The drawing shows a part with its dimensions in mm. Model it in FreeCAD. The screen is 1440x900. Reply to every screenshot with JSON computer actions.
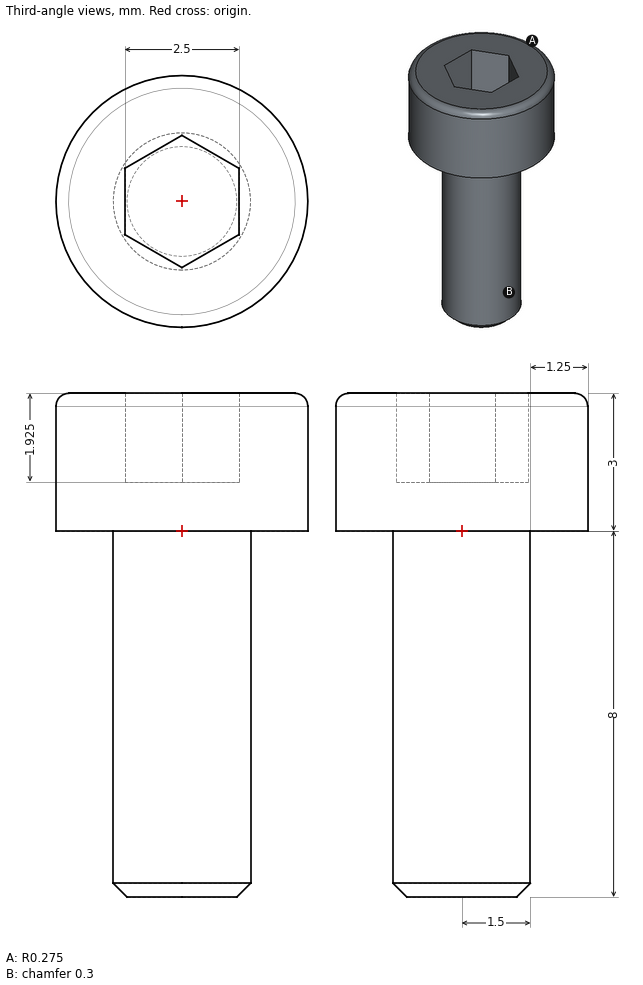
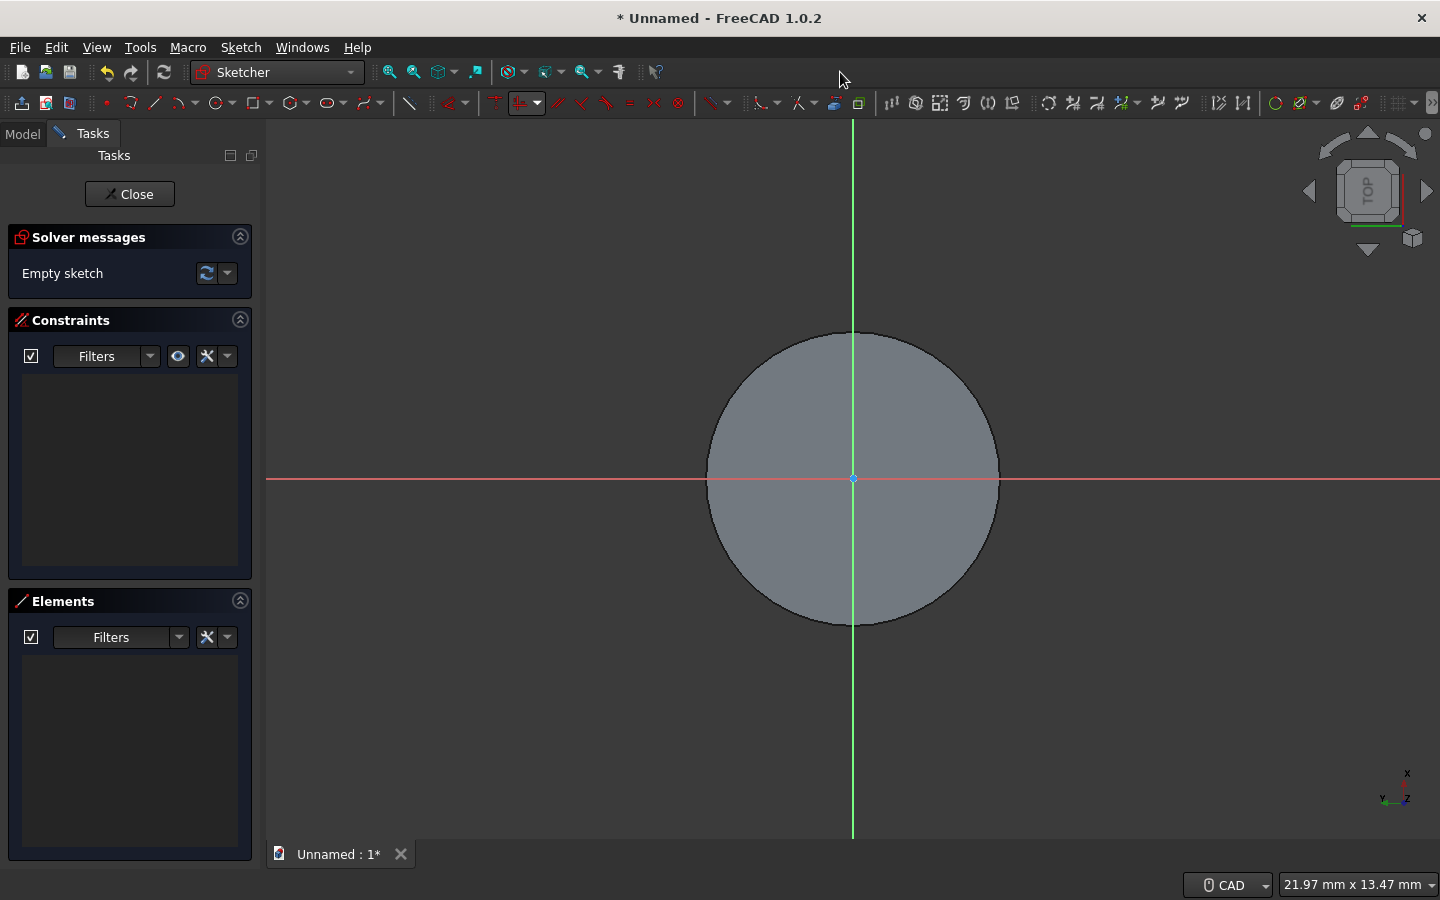
{"action": "scroll", "coordinate": [883, 479], "scroll_direction": "up", "scroll_amount": 6}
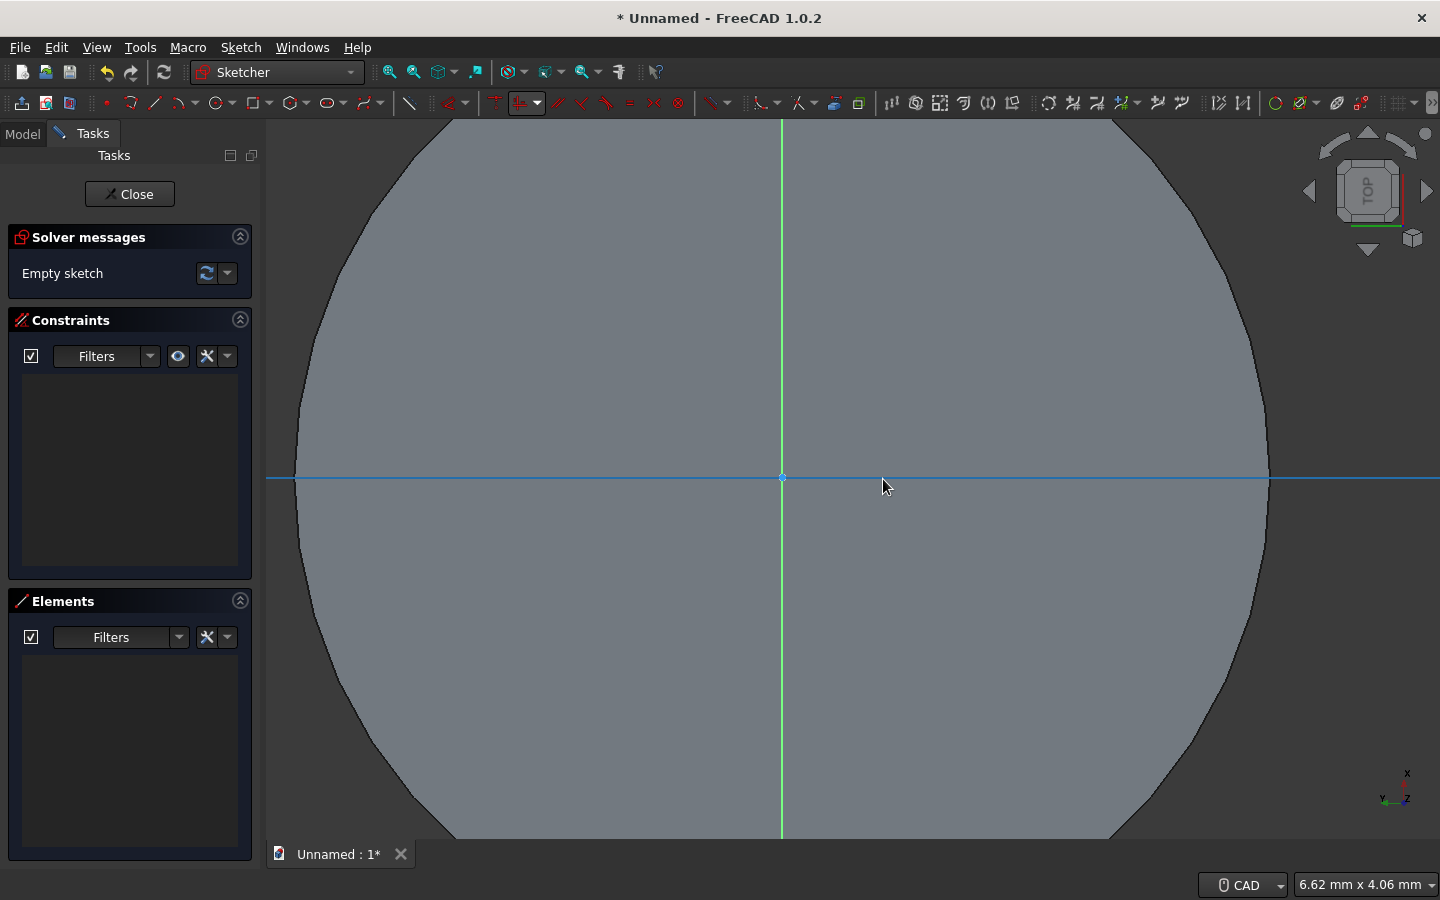
{"action": "left_click", "coordinate": [290, 104]}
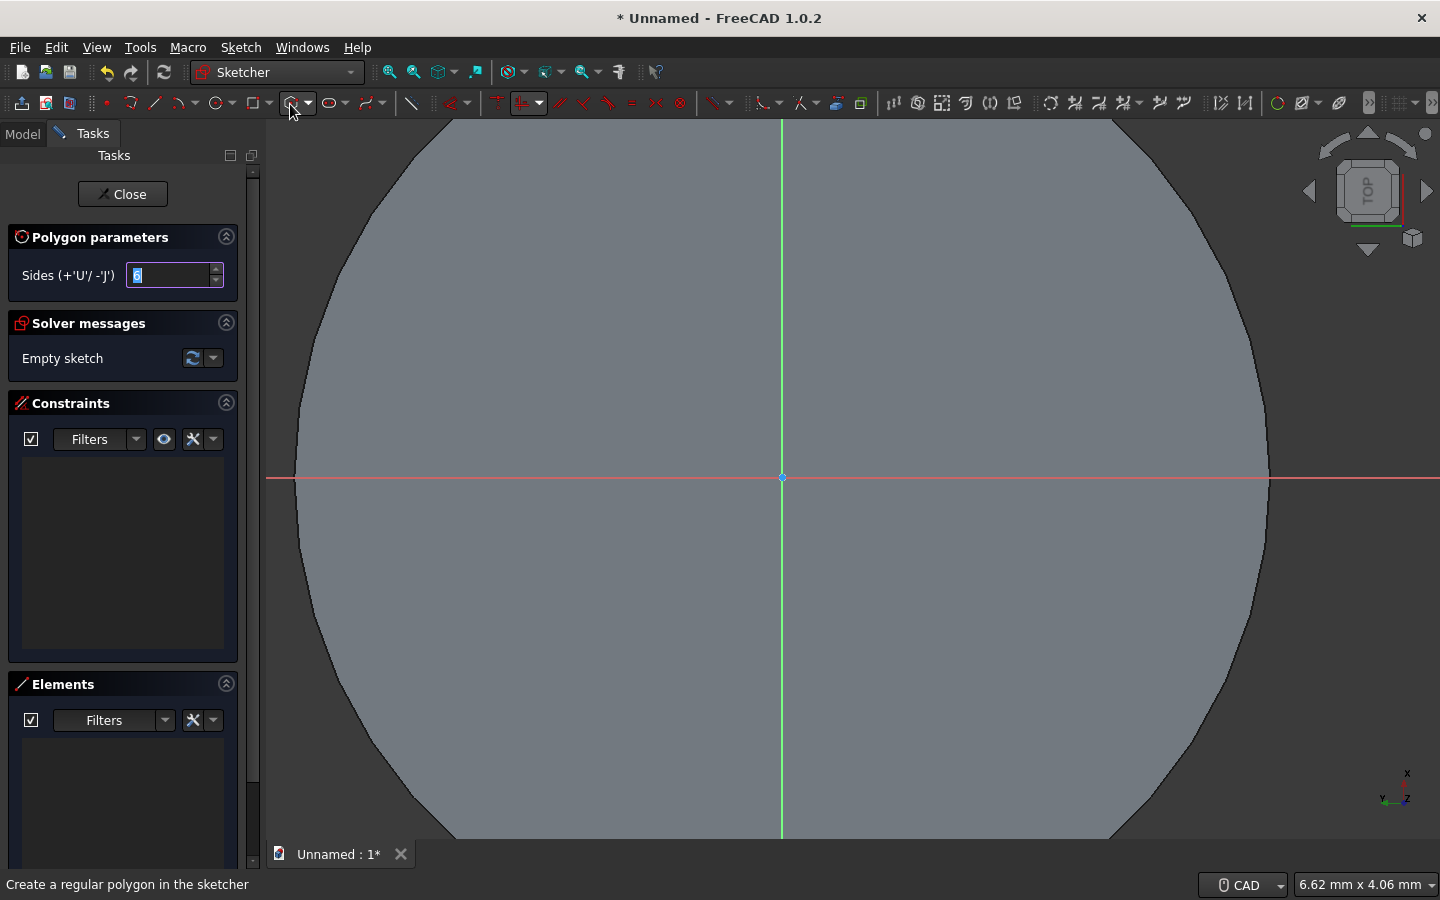
{"action": "left_click", "coordinate": [782, 478]}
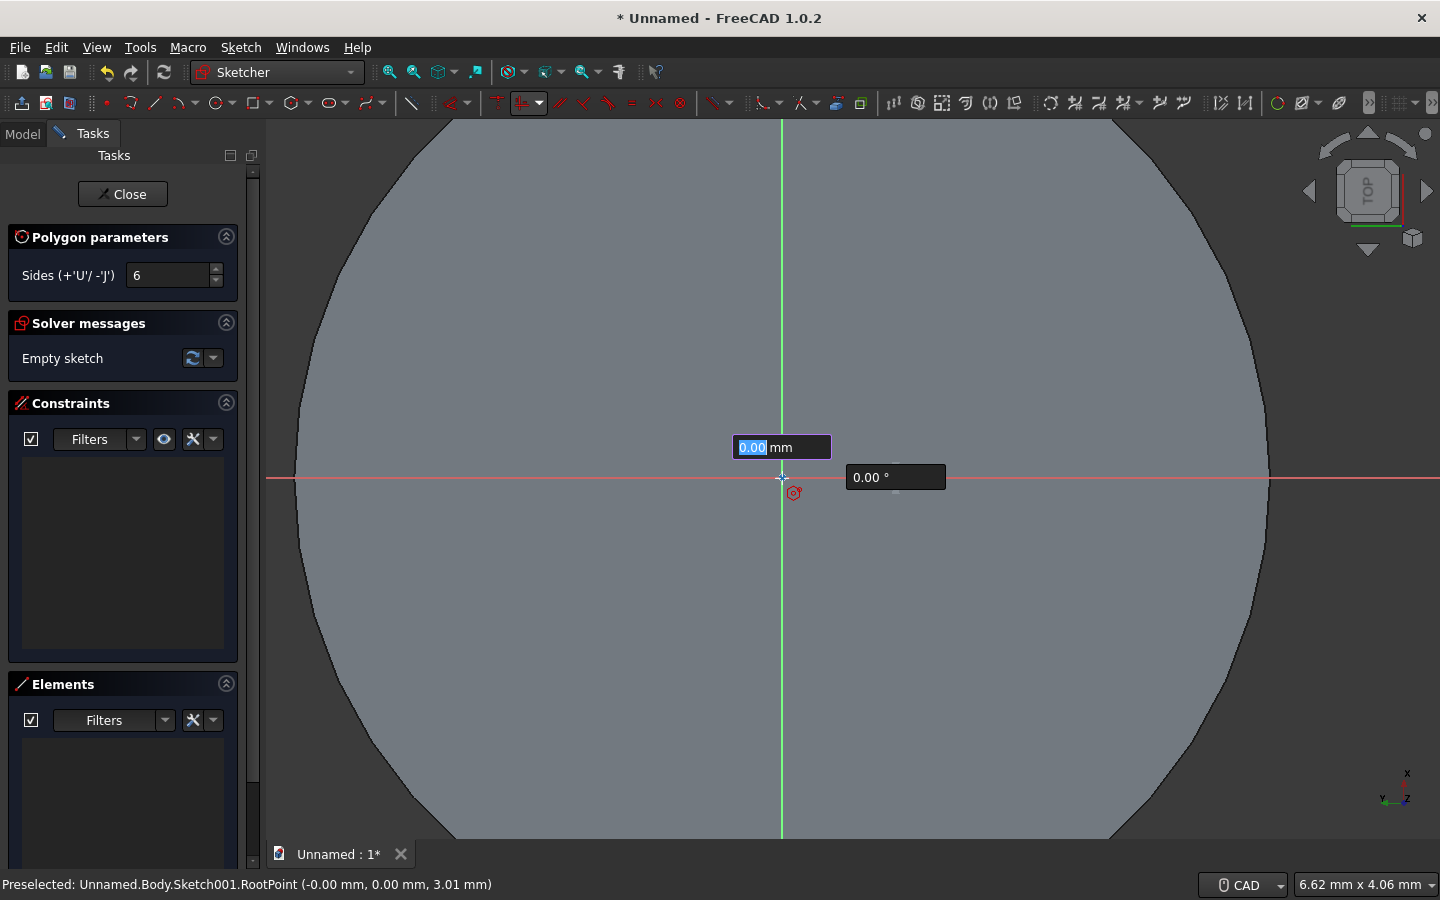
{"action": "left_click", "coordinate": [526, 478]}
{"action": "key", "text": "Escape"}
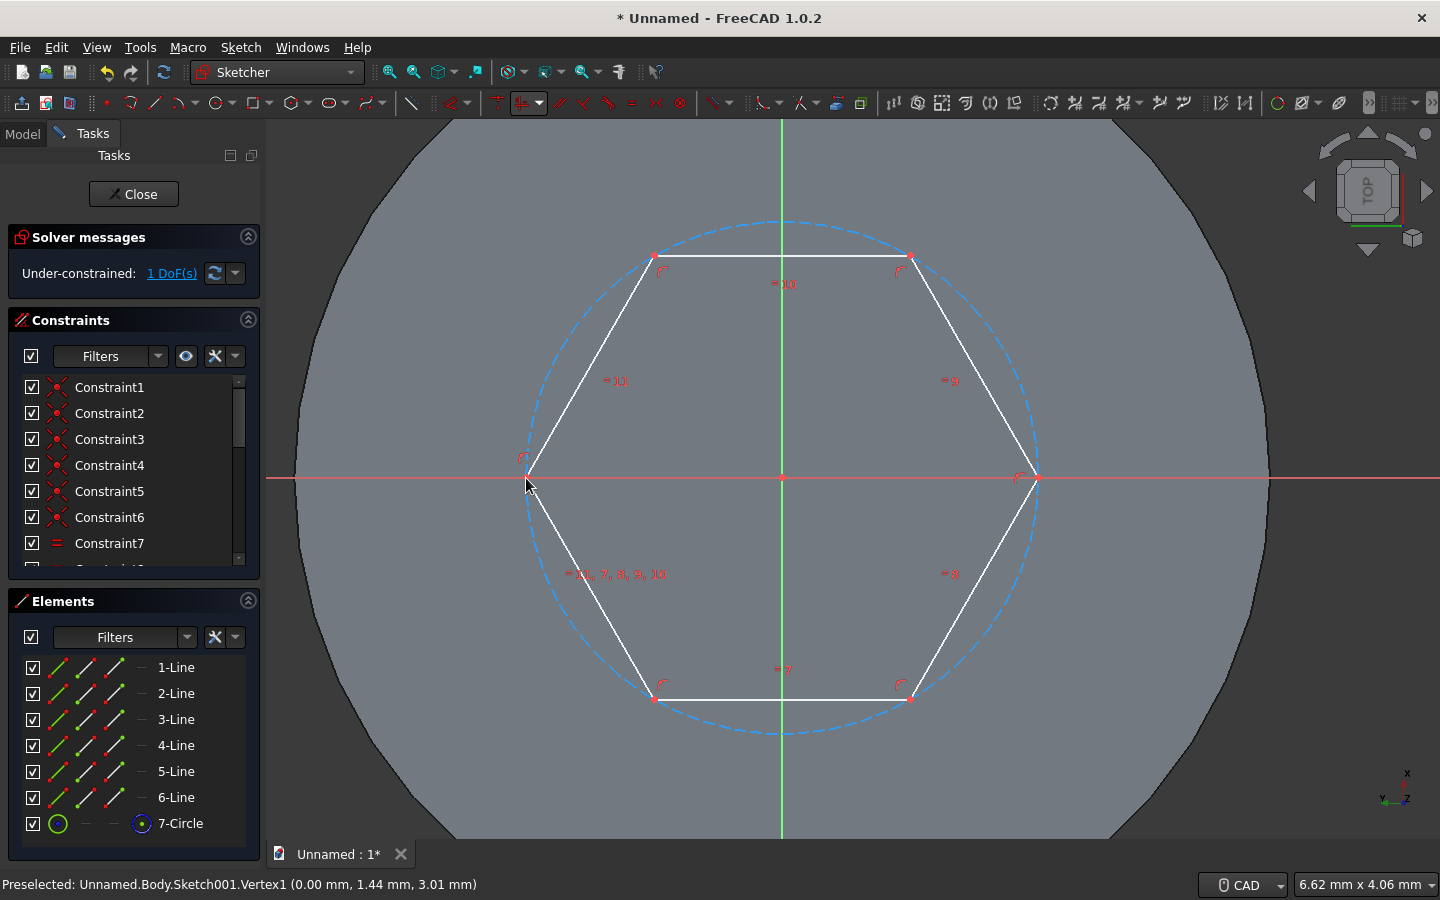
{"action": "left_click", "coordinate": [450, 104]}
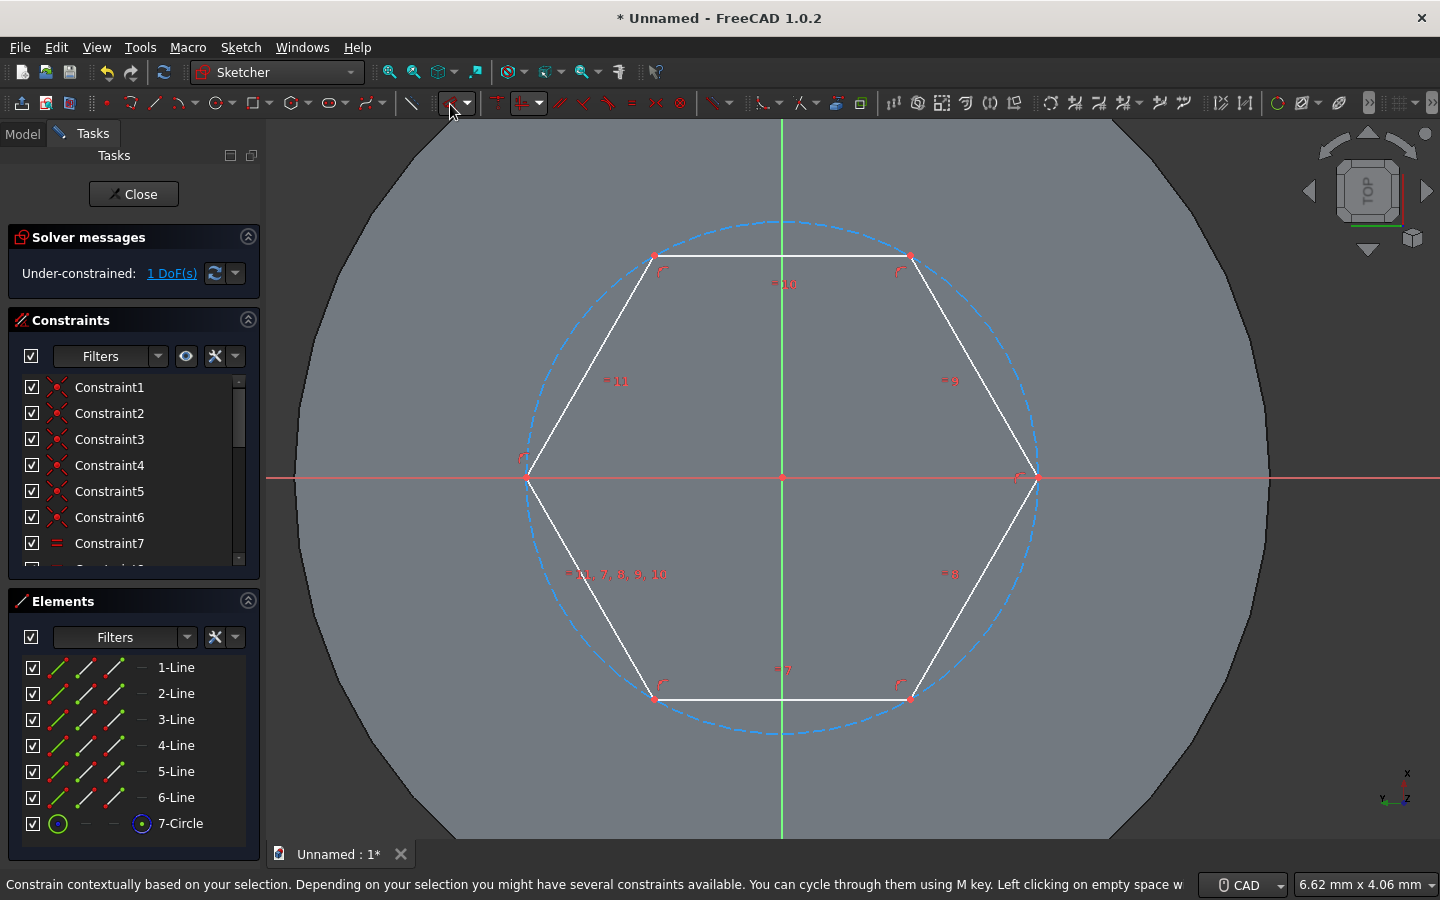
{"action": "left_click", "coordinate": [654, 700]}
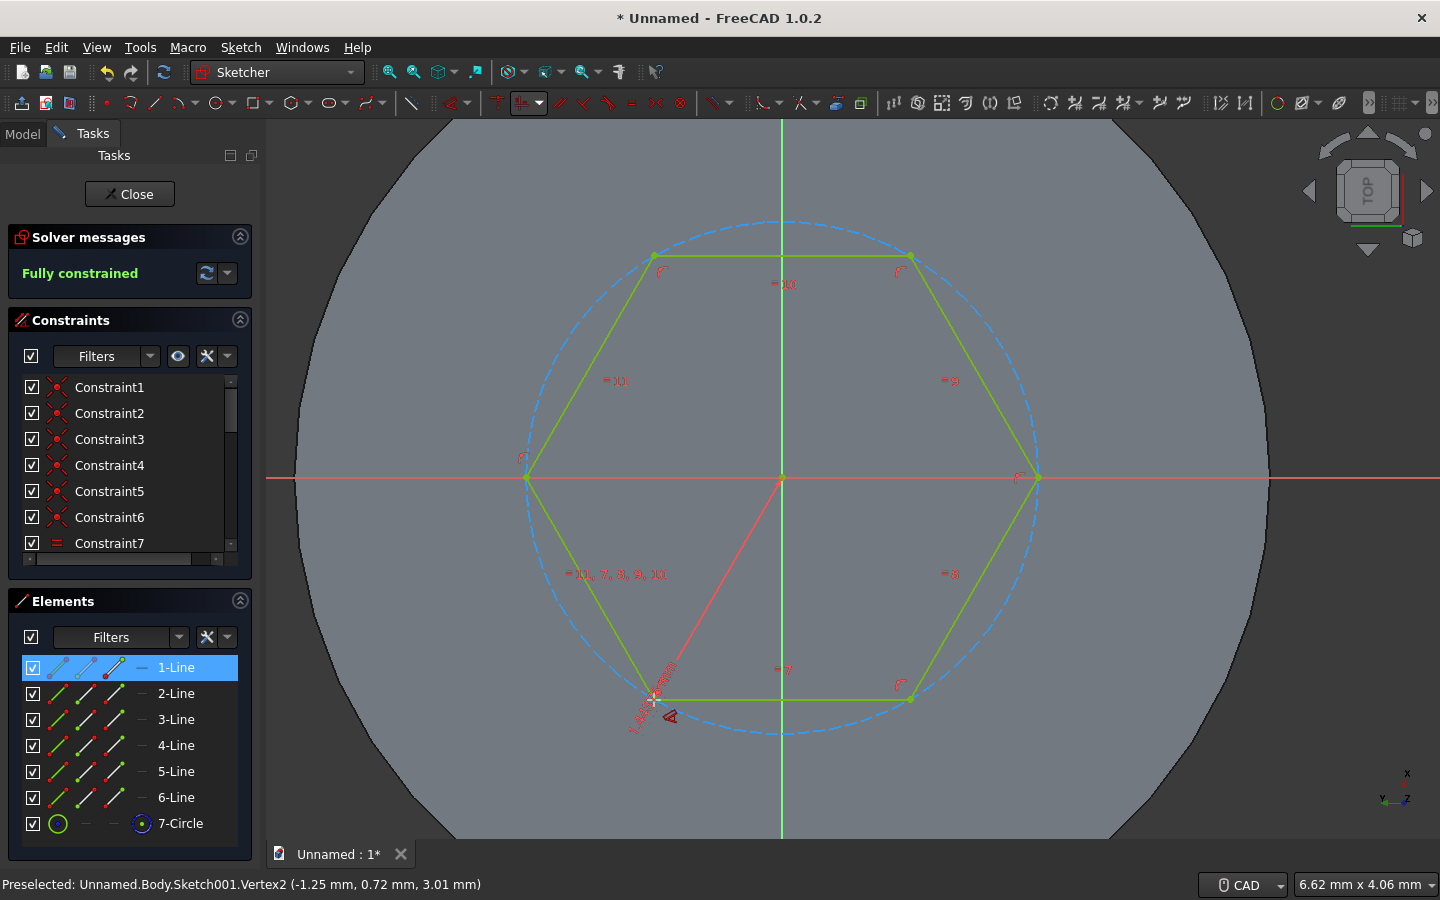
{"action": "left_click", "coordinate": [910, 256]}
{"action": "left_click", "coordinate": [944, 376]}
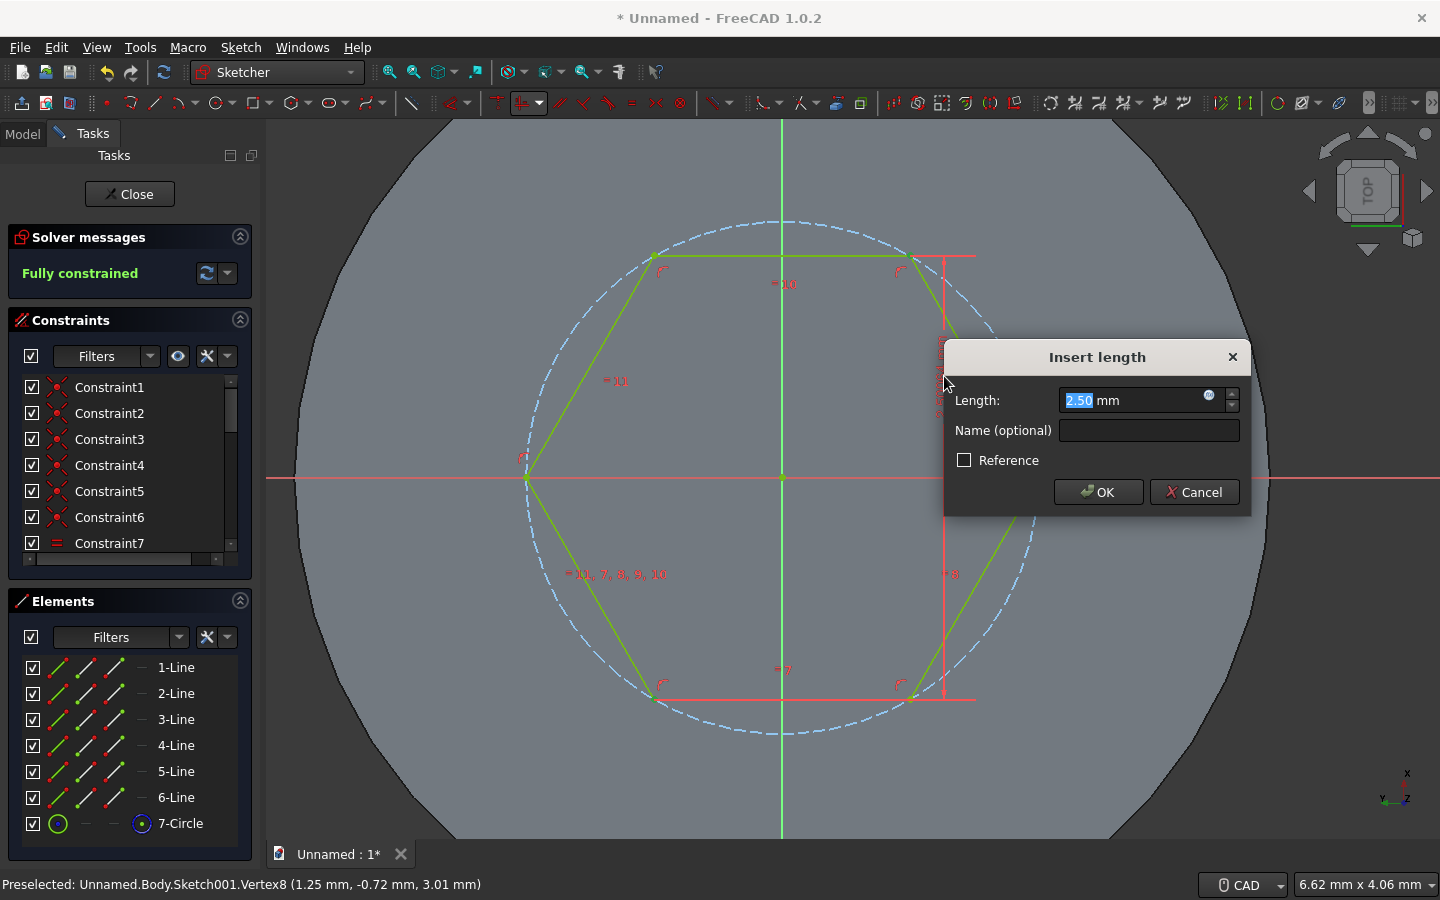
{"action": "type", "text": "2.5"}
{"action": "key", "text": "Return"}
{"action": "key", "text": "Escape"}